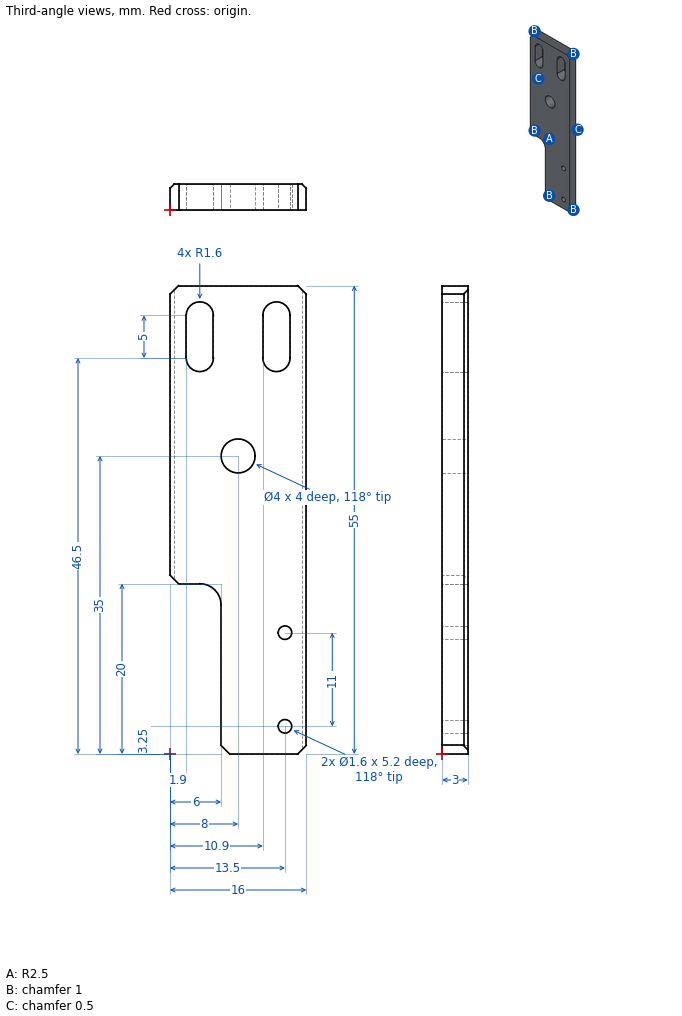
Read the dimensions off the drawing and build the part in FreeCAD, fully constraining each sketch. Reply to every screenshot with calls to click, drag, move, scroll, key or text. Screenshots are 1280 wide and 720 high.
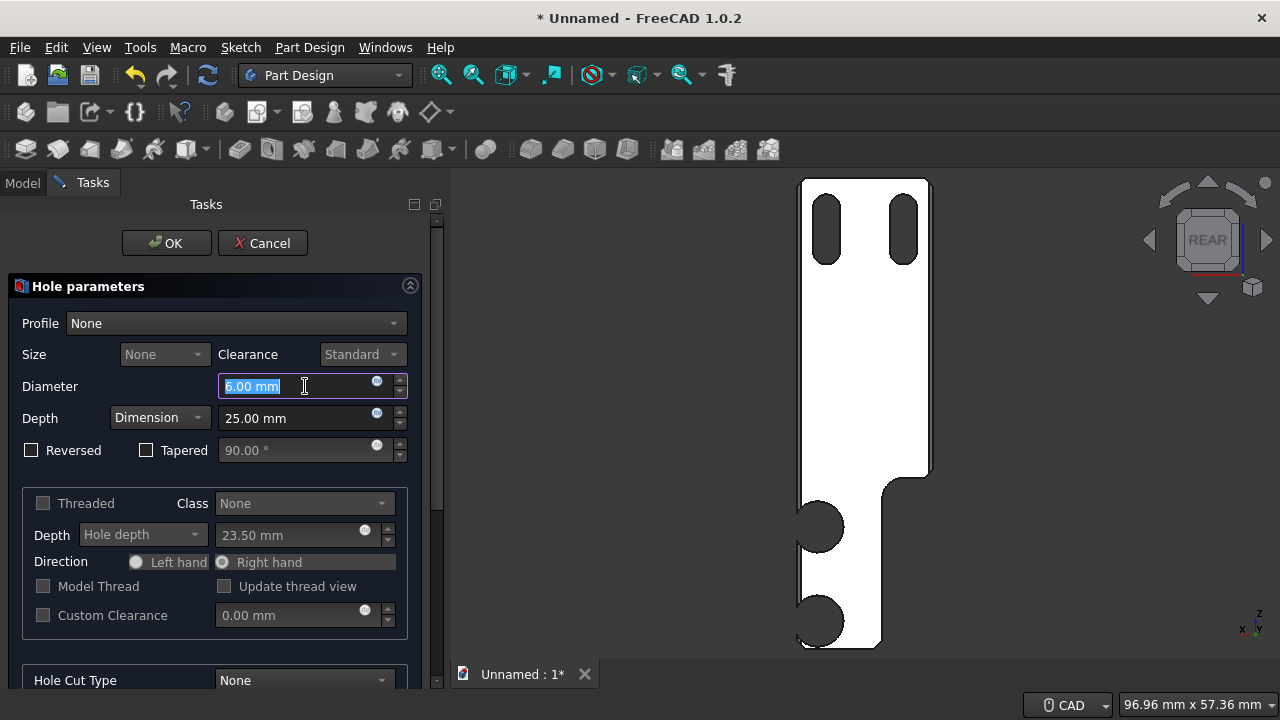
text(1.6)
key(Tab)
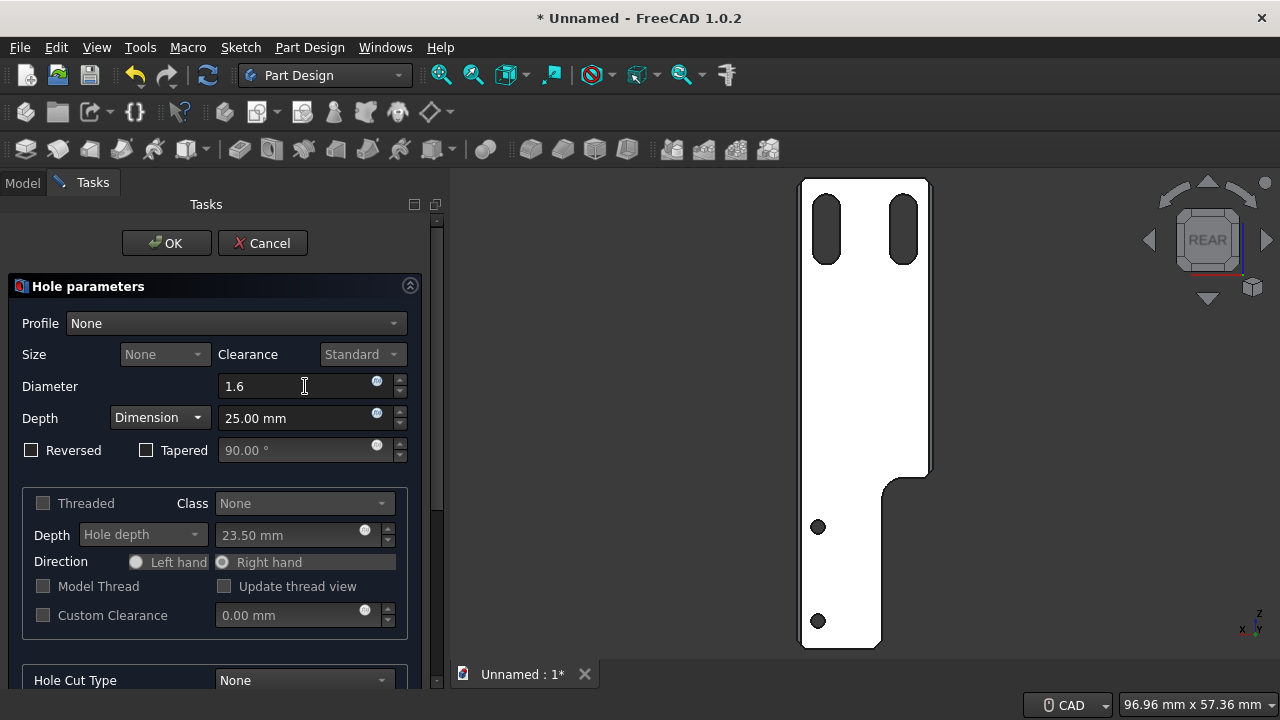
triple_click(305, 418)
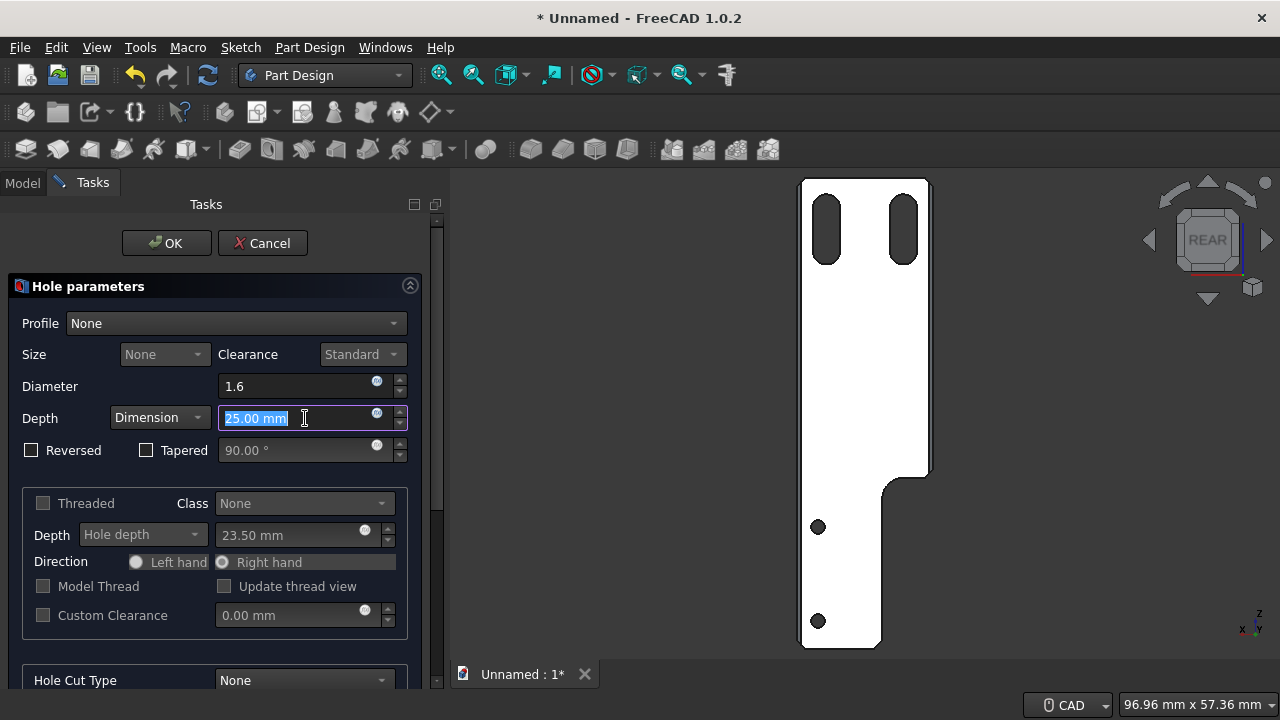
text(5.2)
key(Tab)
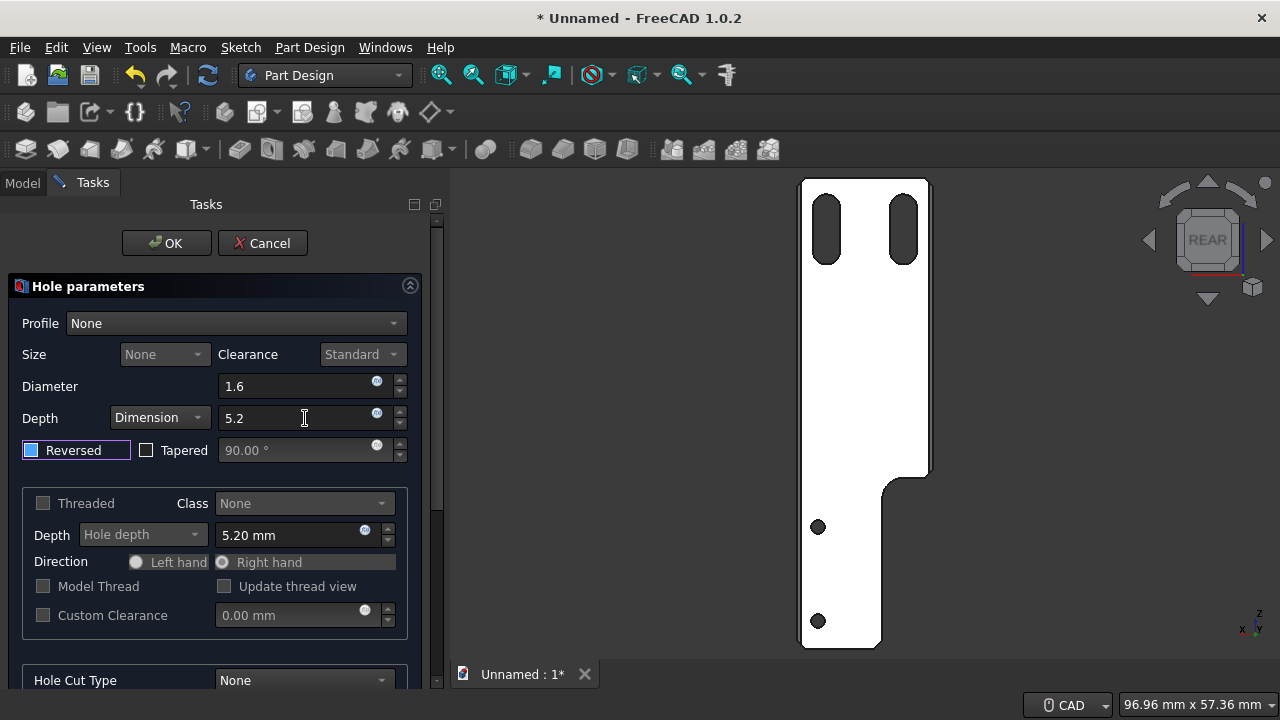
click(167, 243)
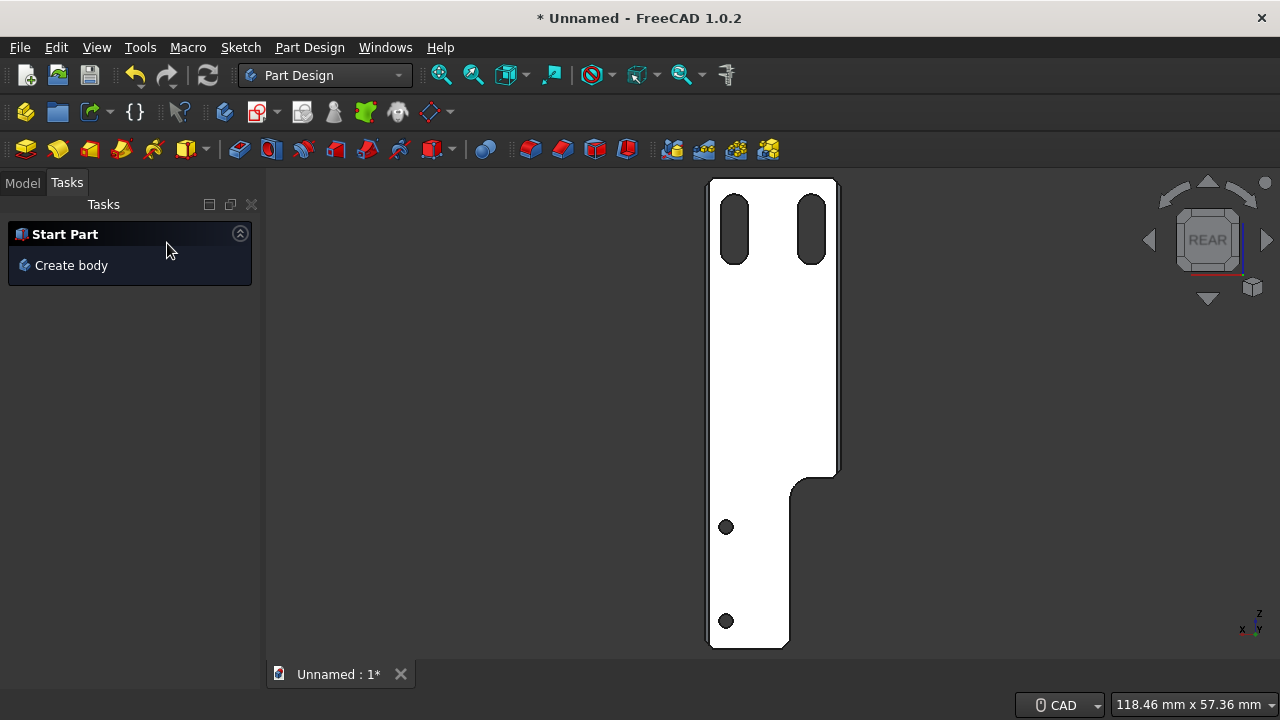
click(258, 112)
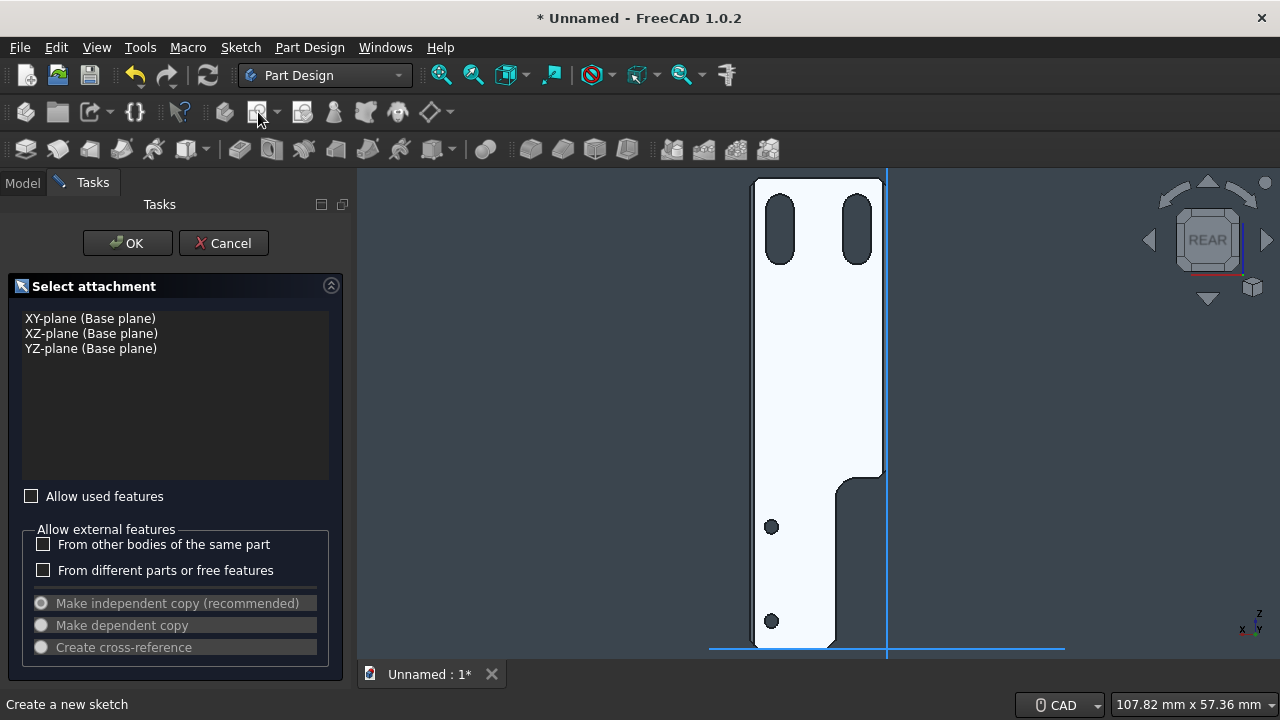
click(82, 334)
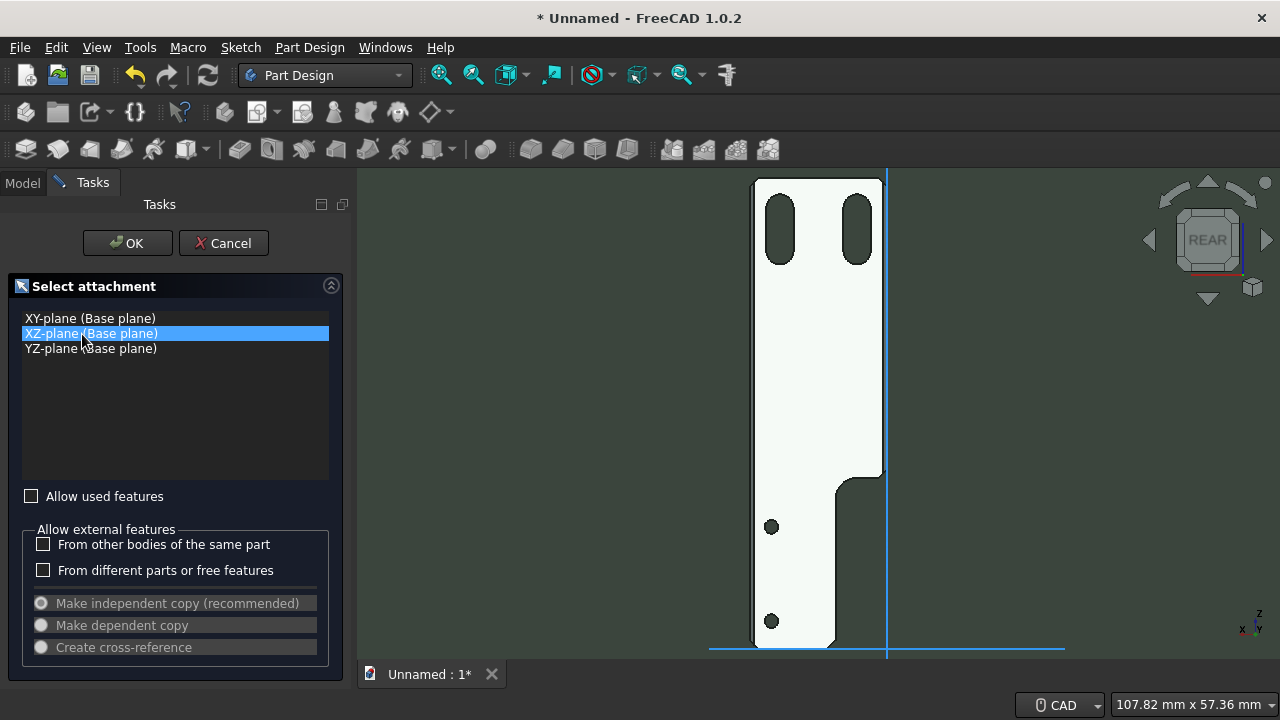
click(128, 243)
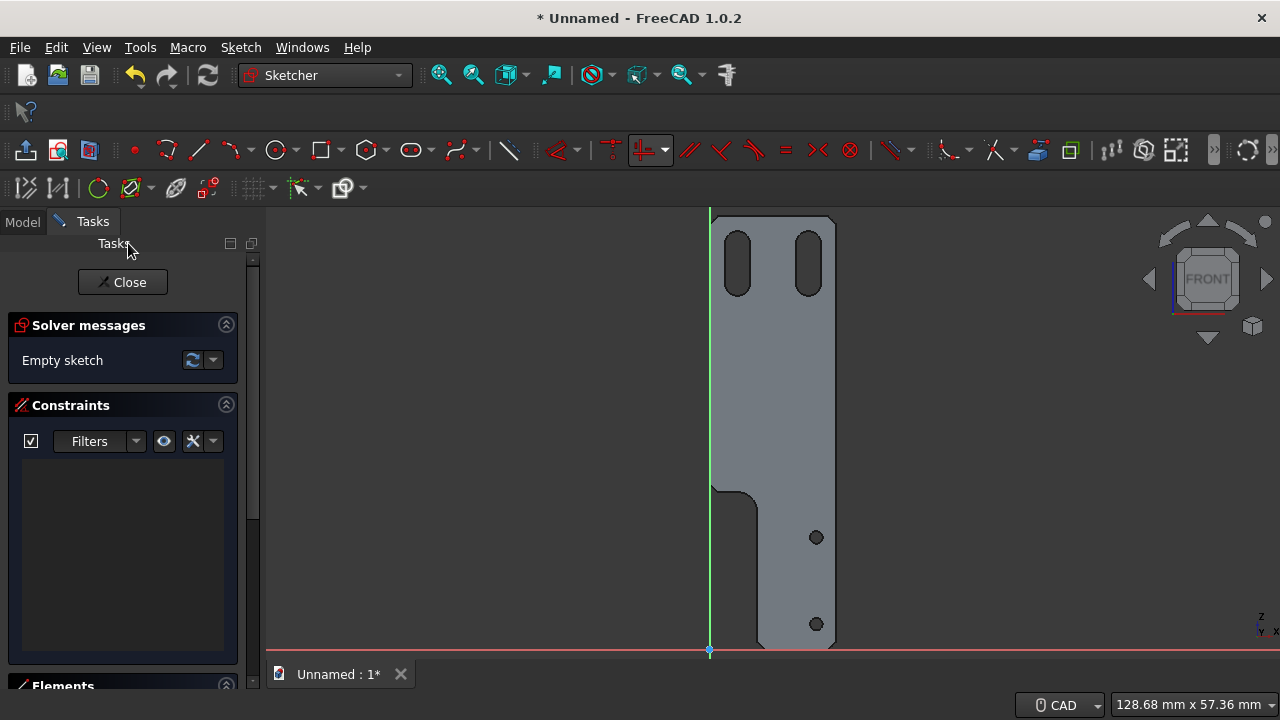
scroll(782, 367, up, 11)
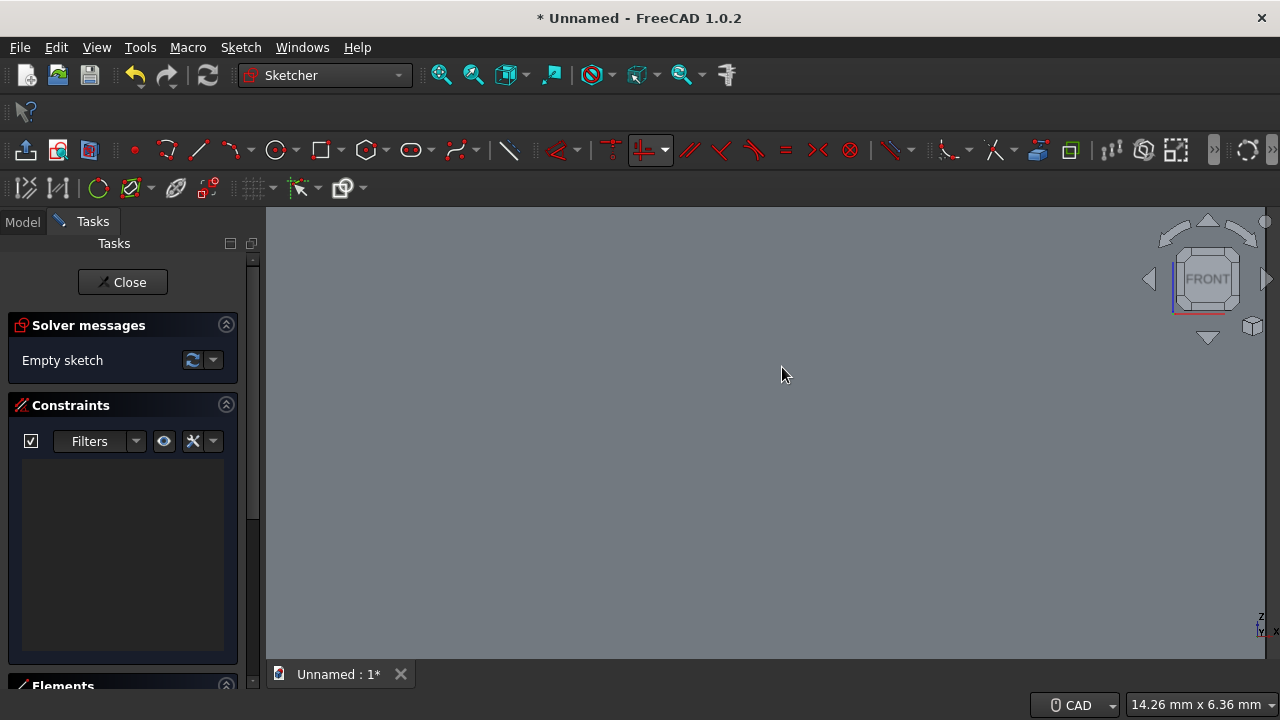
click(276, 150)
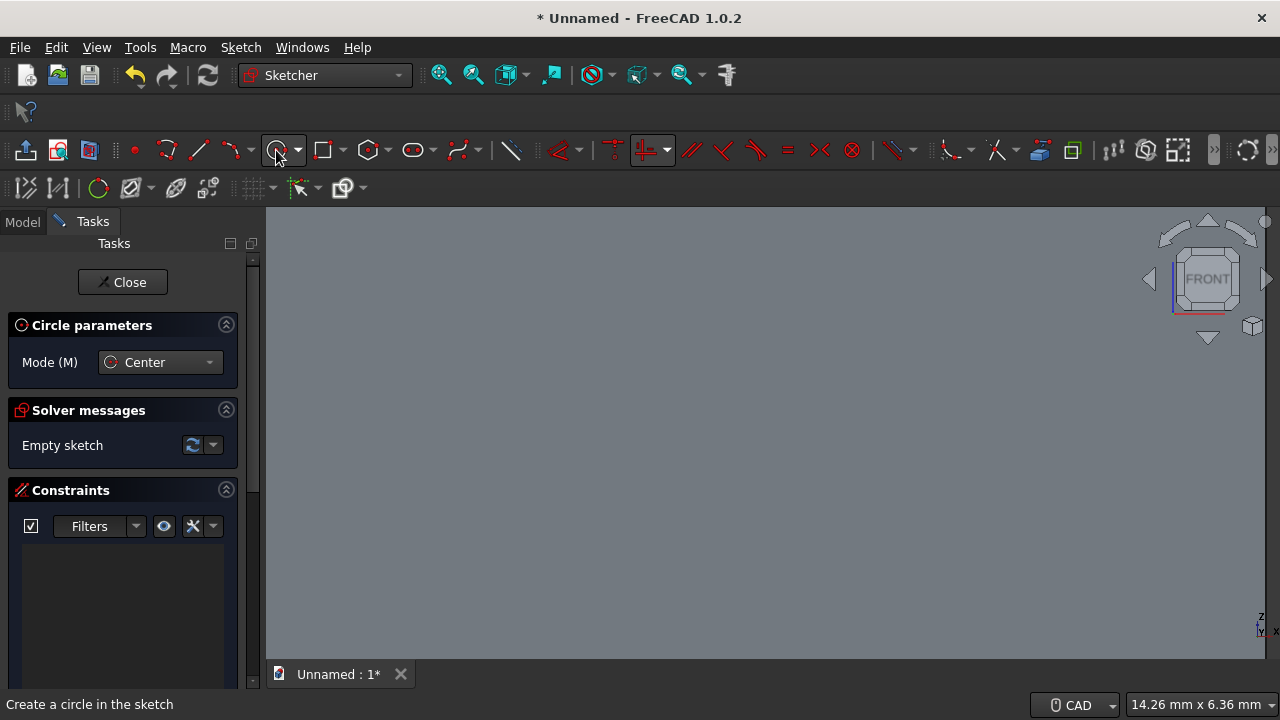
click(697, 426)
move(797, 326)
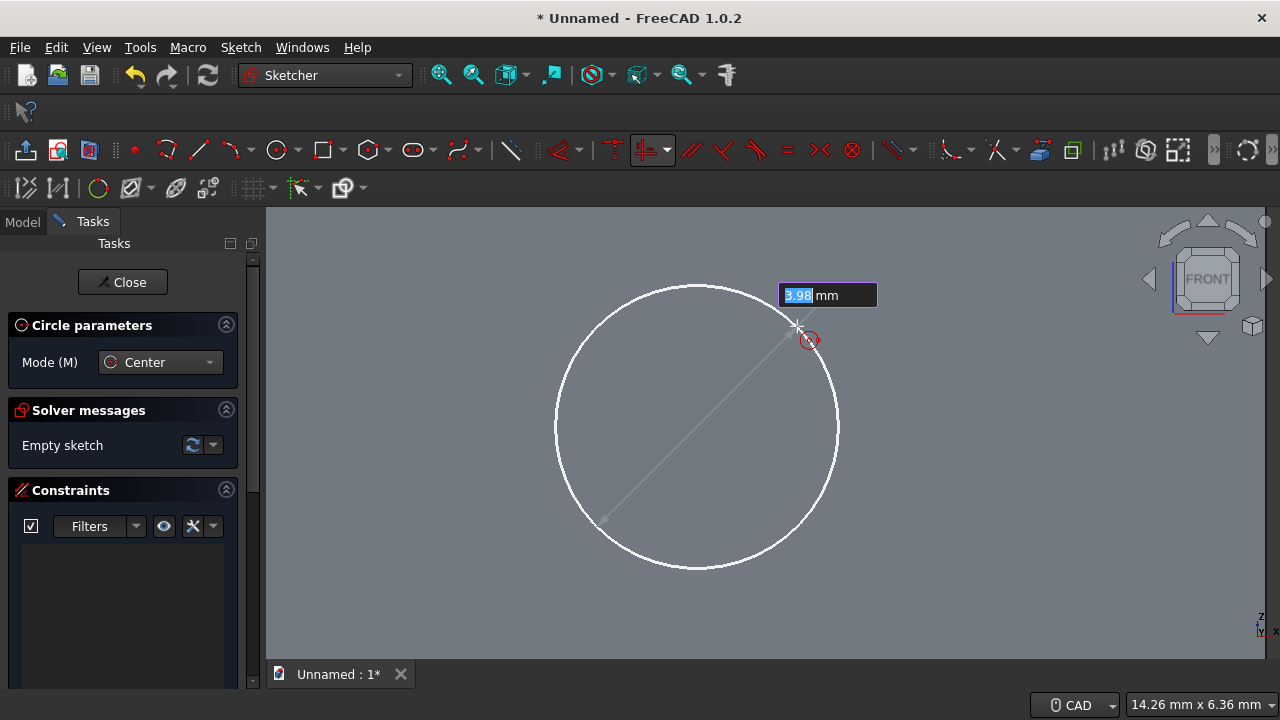
text(4)
key(Return)
key(Escape)